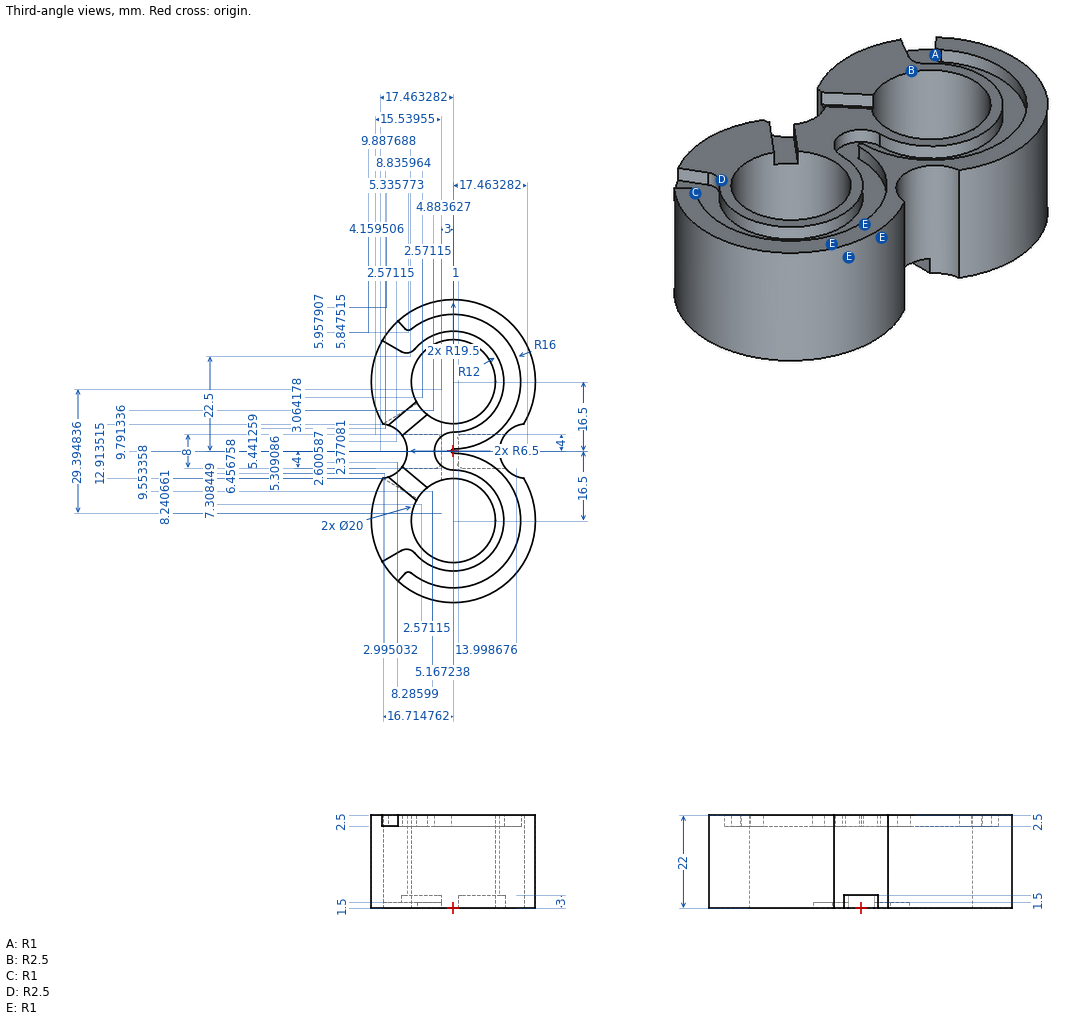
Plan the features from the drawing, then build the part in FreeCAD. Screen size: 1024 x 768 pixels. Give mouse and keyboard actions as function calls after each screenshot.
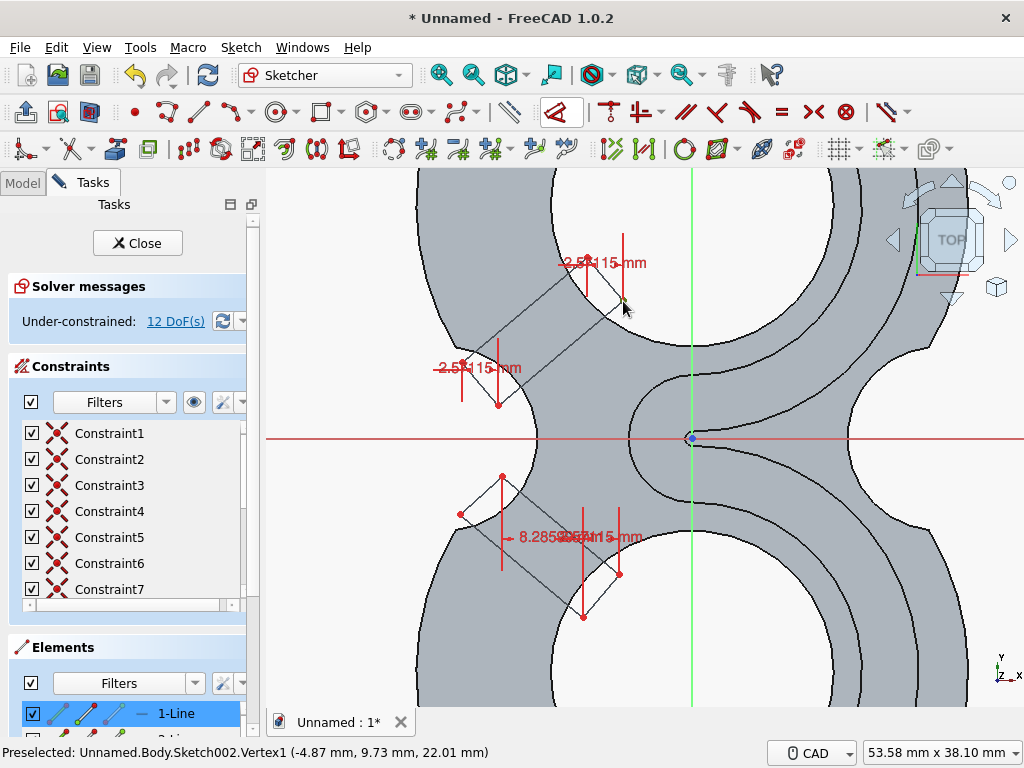
key(l)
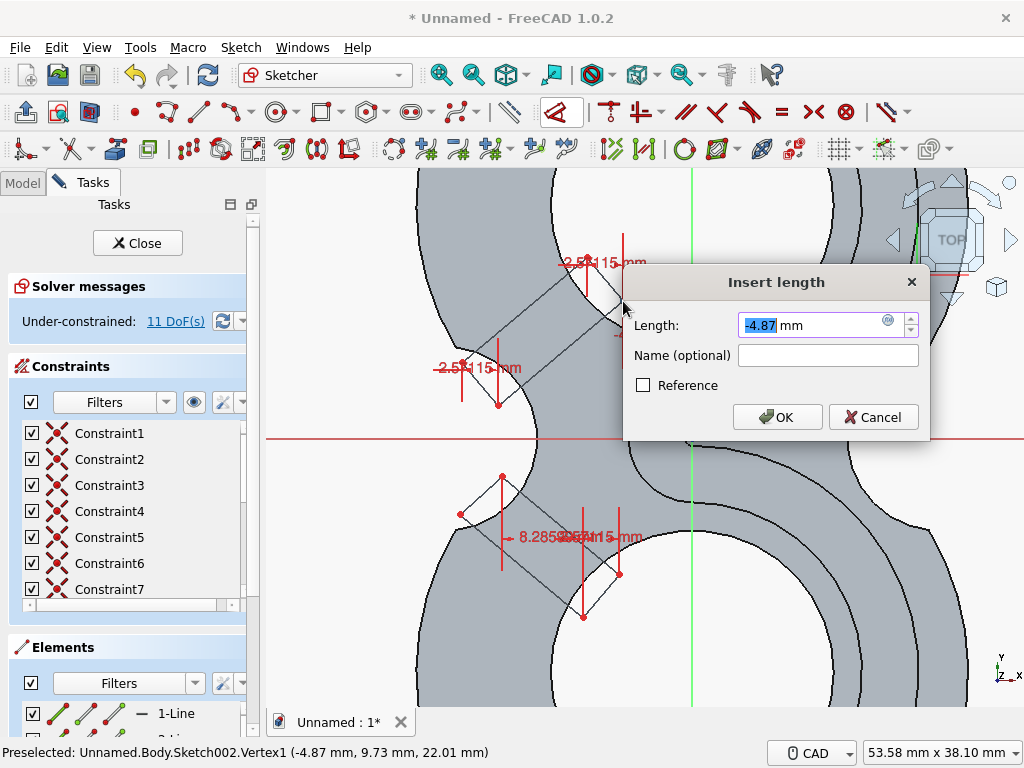
text(-4.883627)
key(Return)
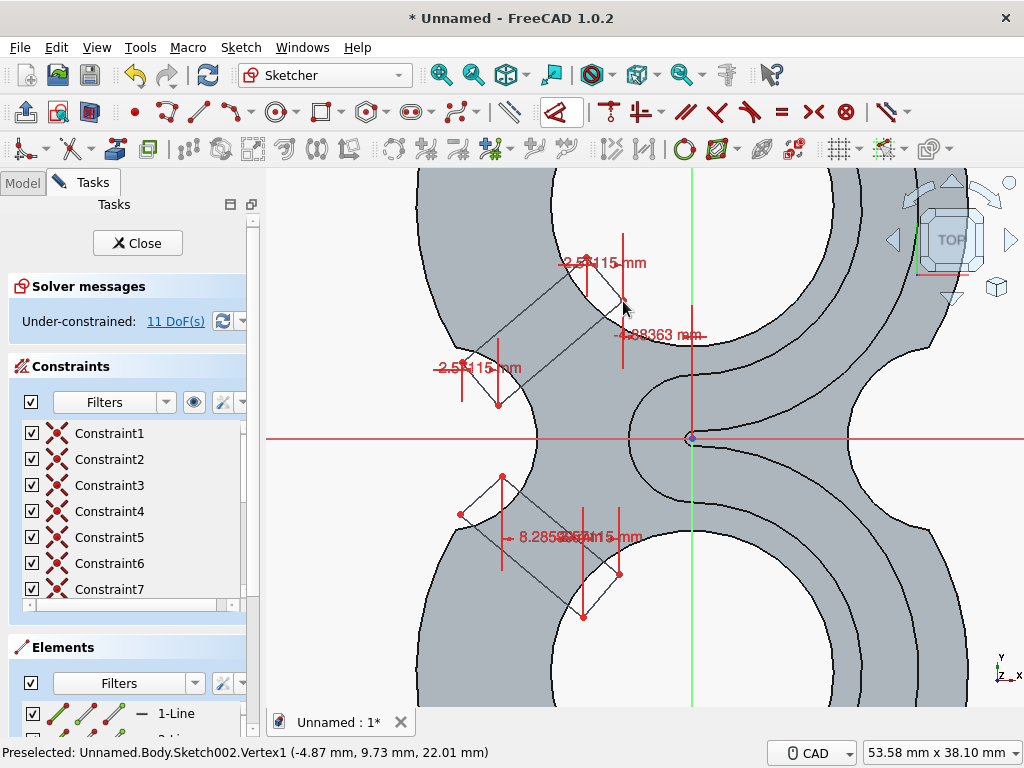
click(623, 301)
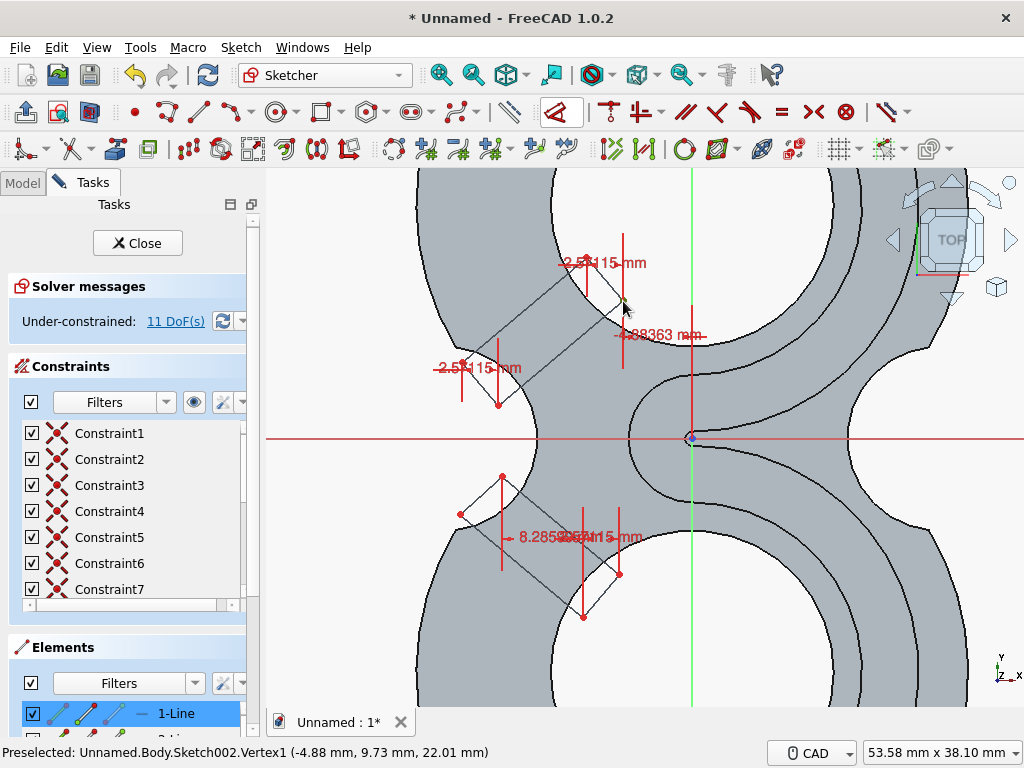
key(i)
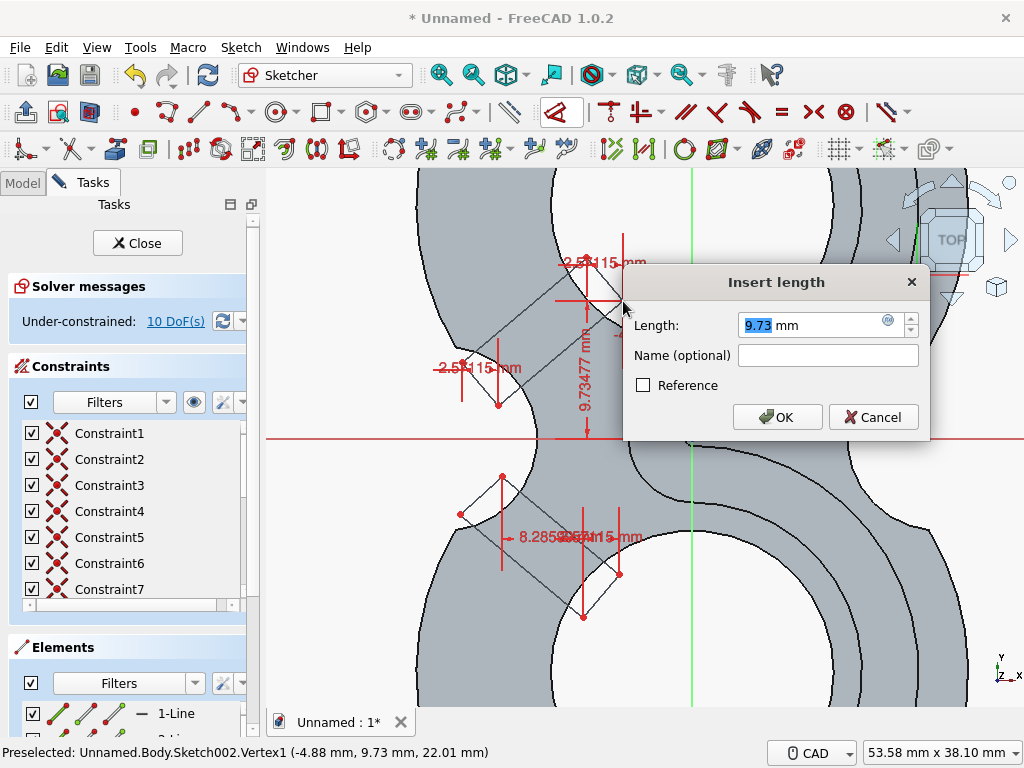
text(9.791336)
key(Return)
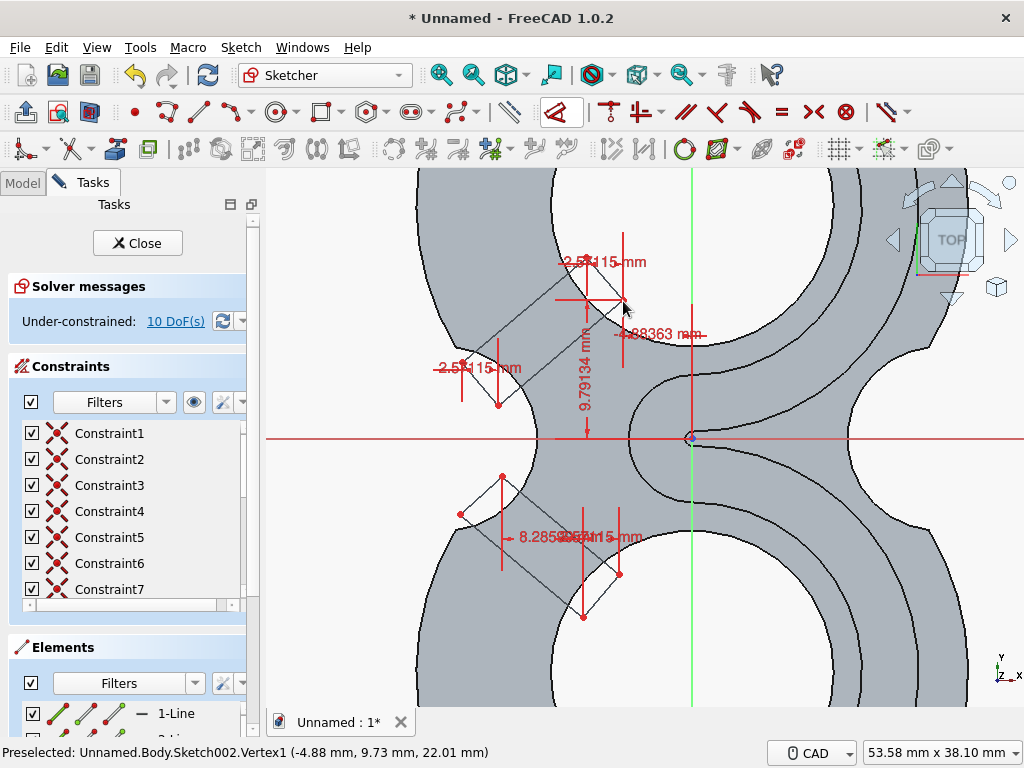
click(462, 363)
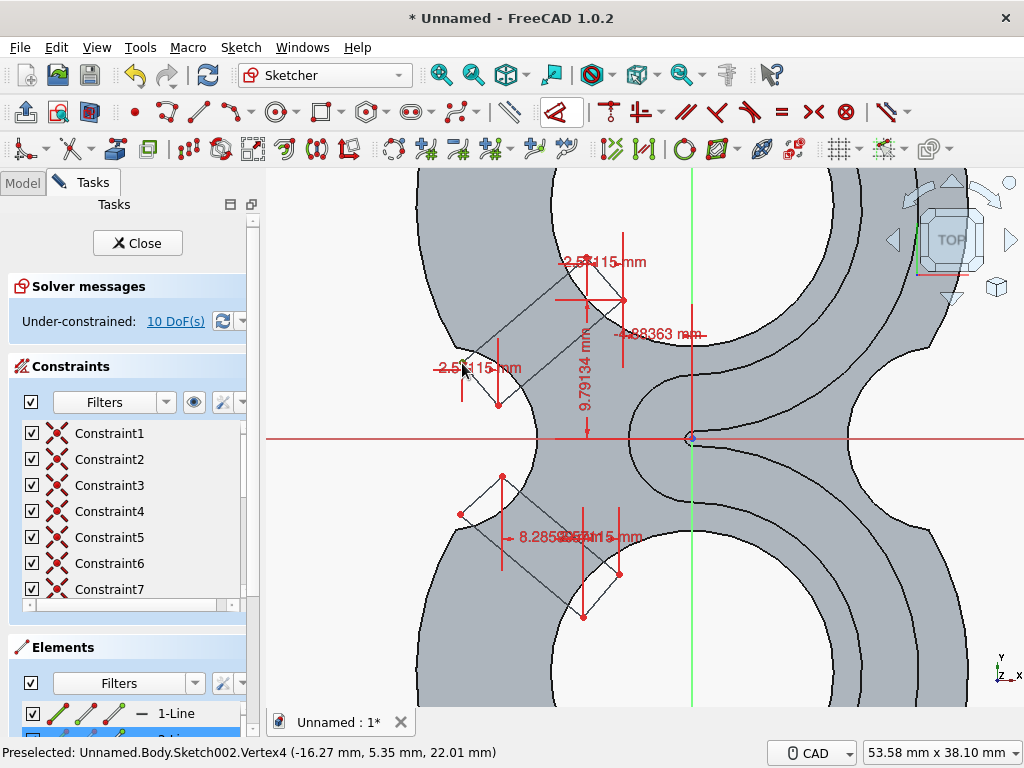
key(i)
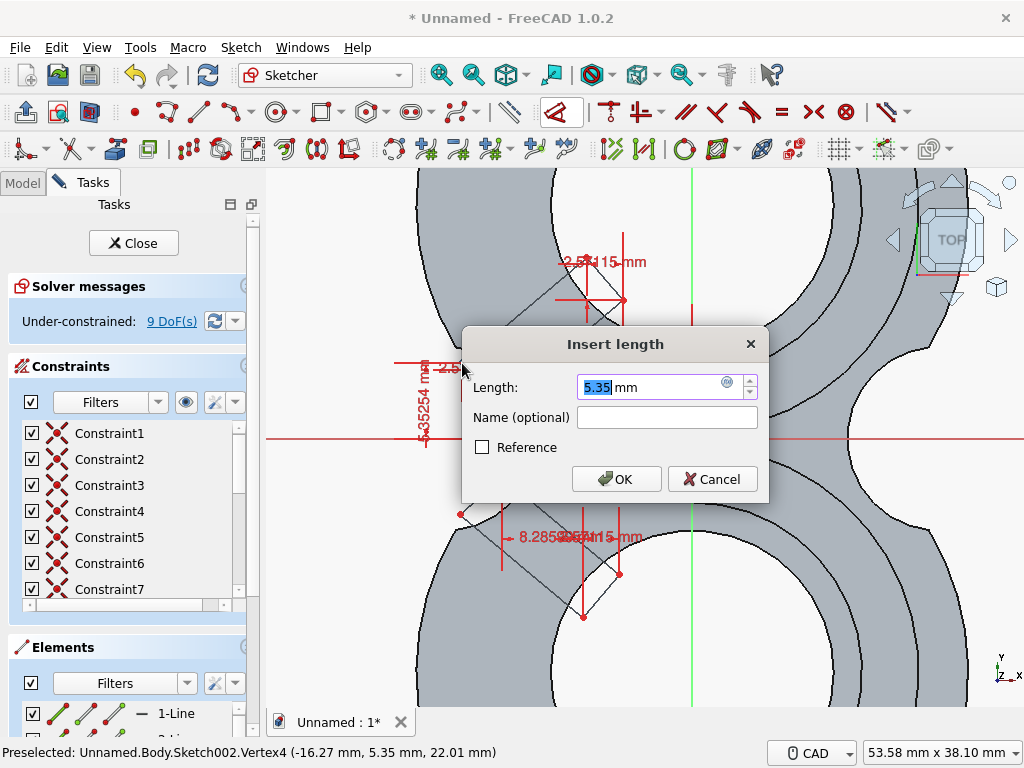
text(5.441259)
key(Return)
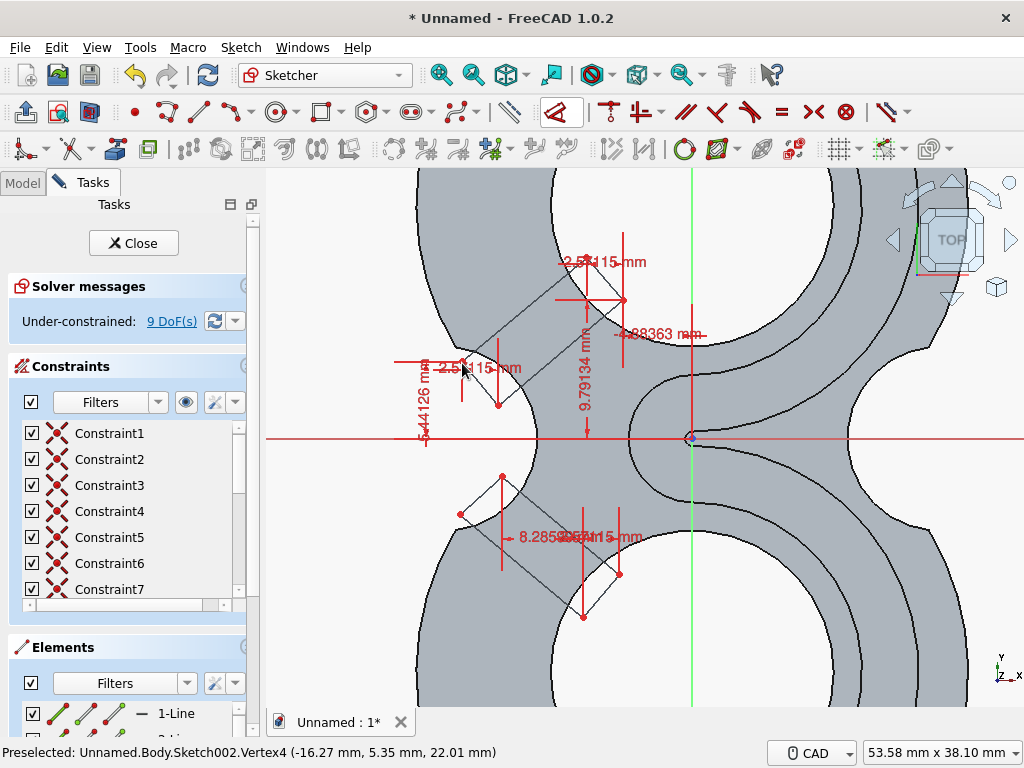
click(498, 406)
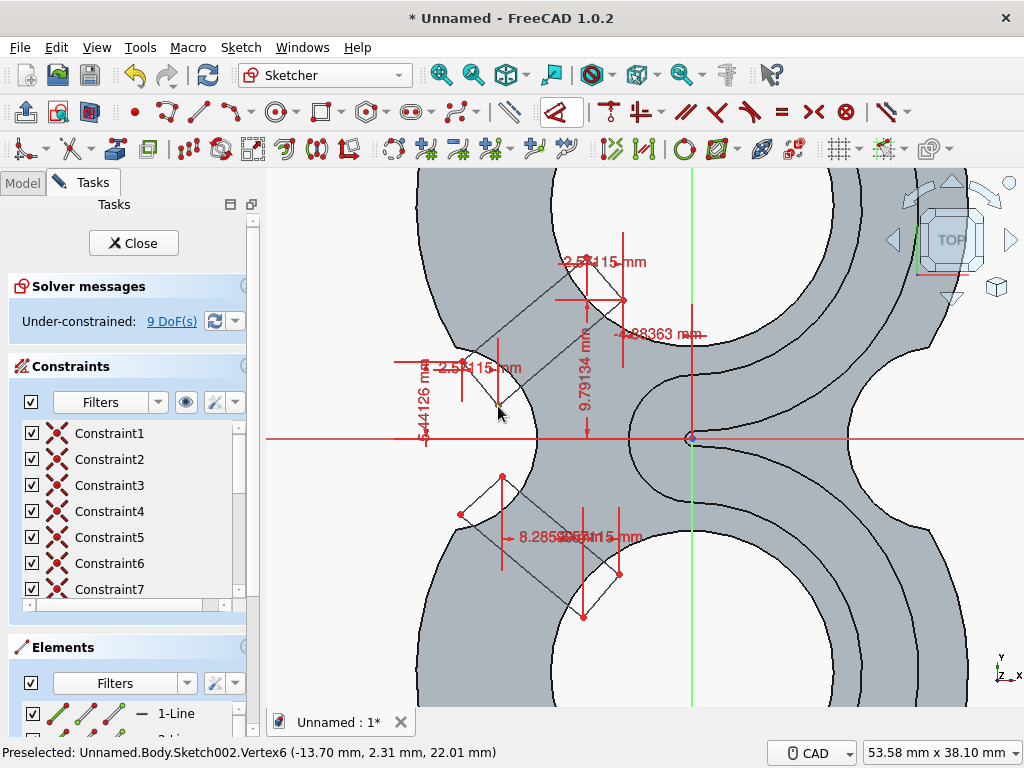
key(i)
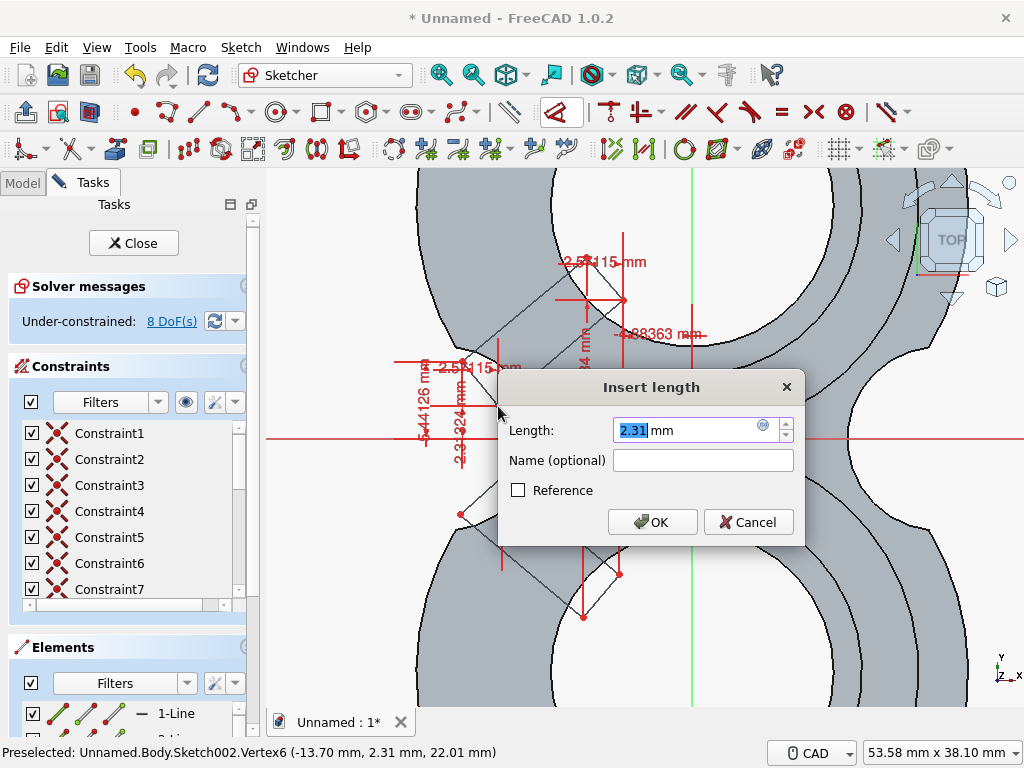
text(2.377081)
key(Return)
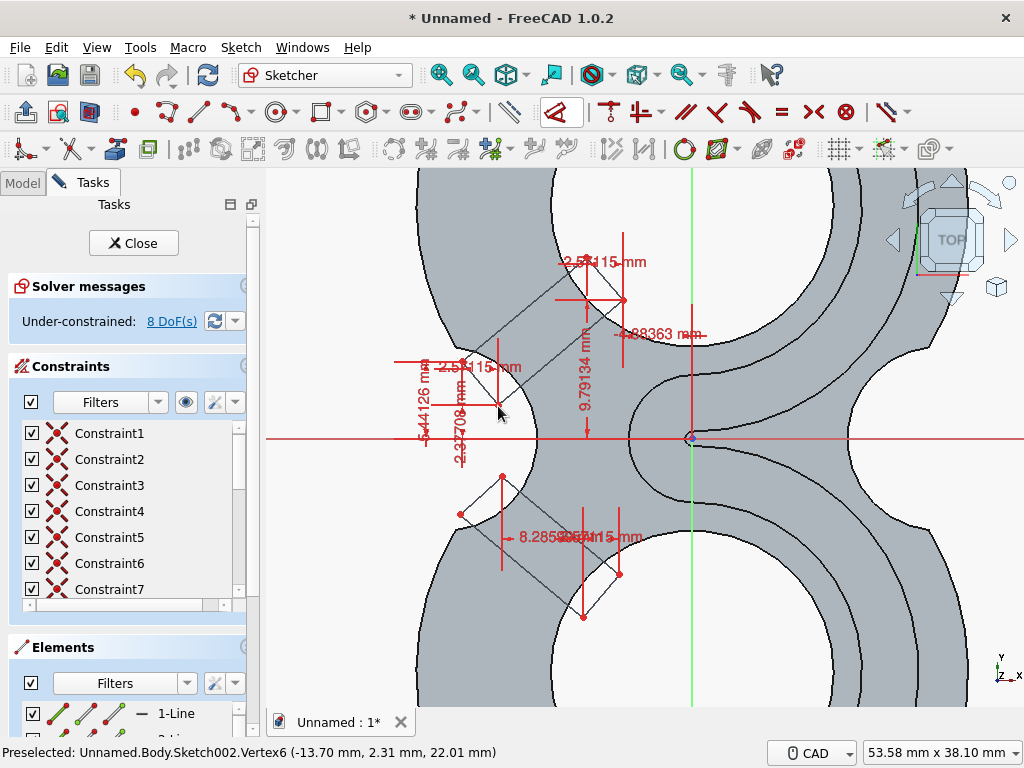
click(619, 575)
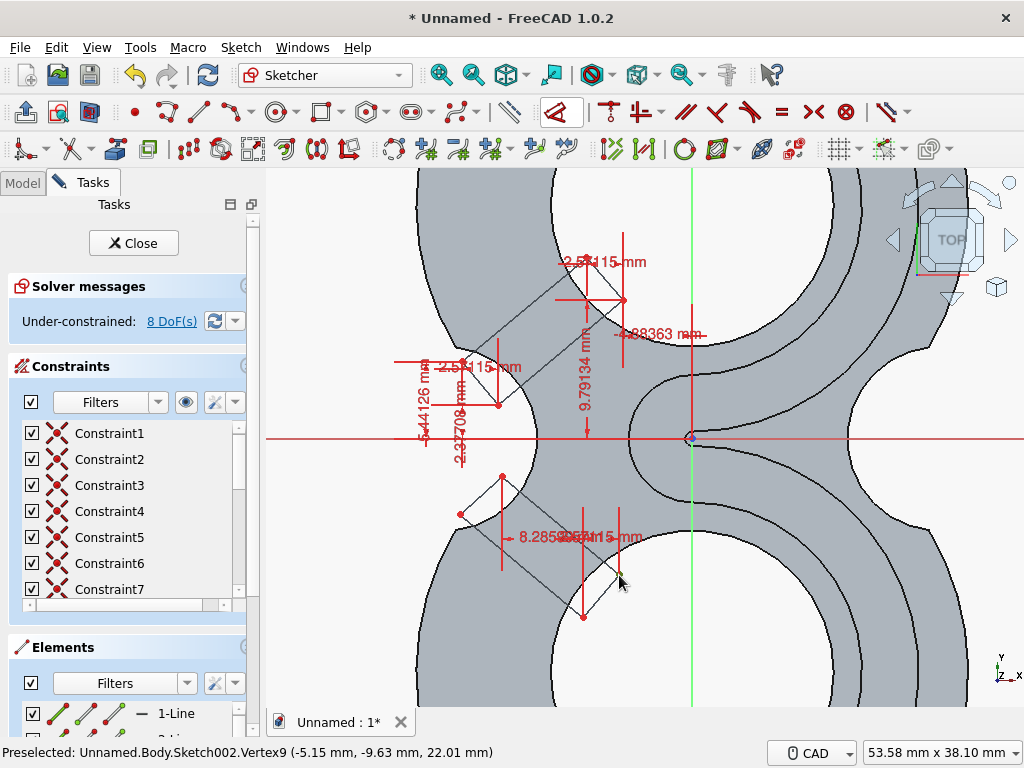
click(578, 112)